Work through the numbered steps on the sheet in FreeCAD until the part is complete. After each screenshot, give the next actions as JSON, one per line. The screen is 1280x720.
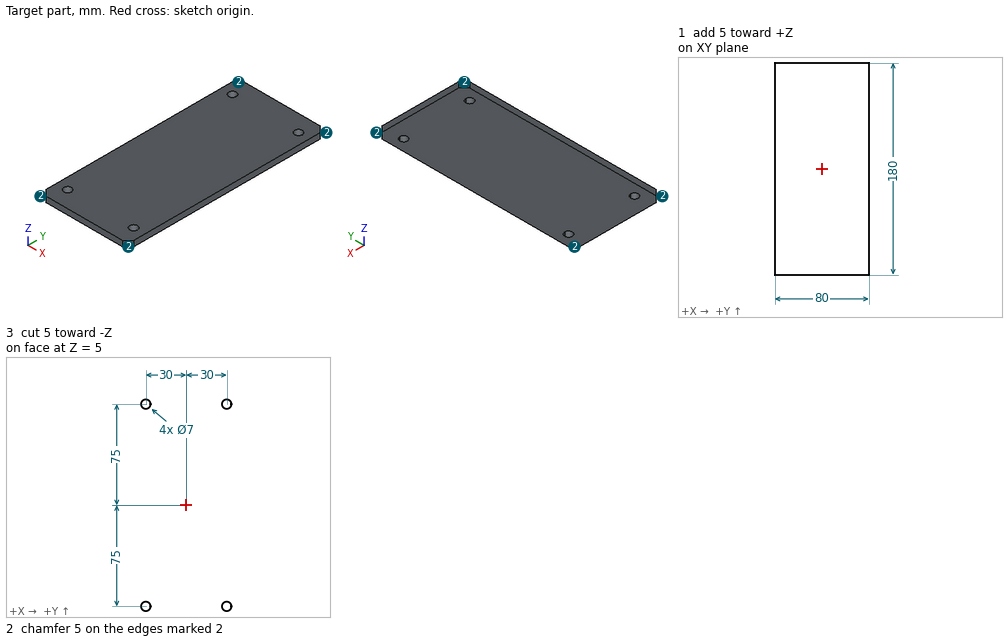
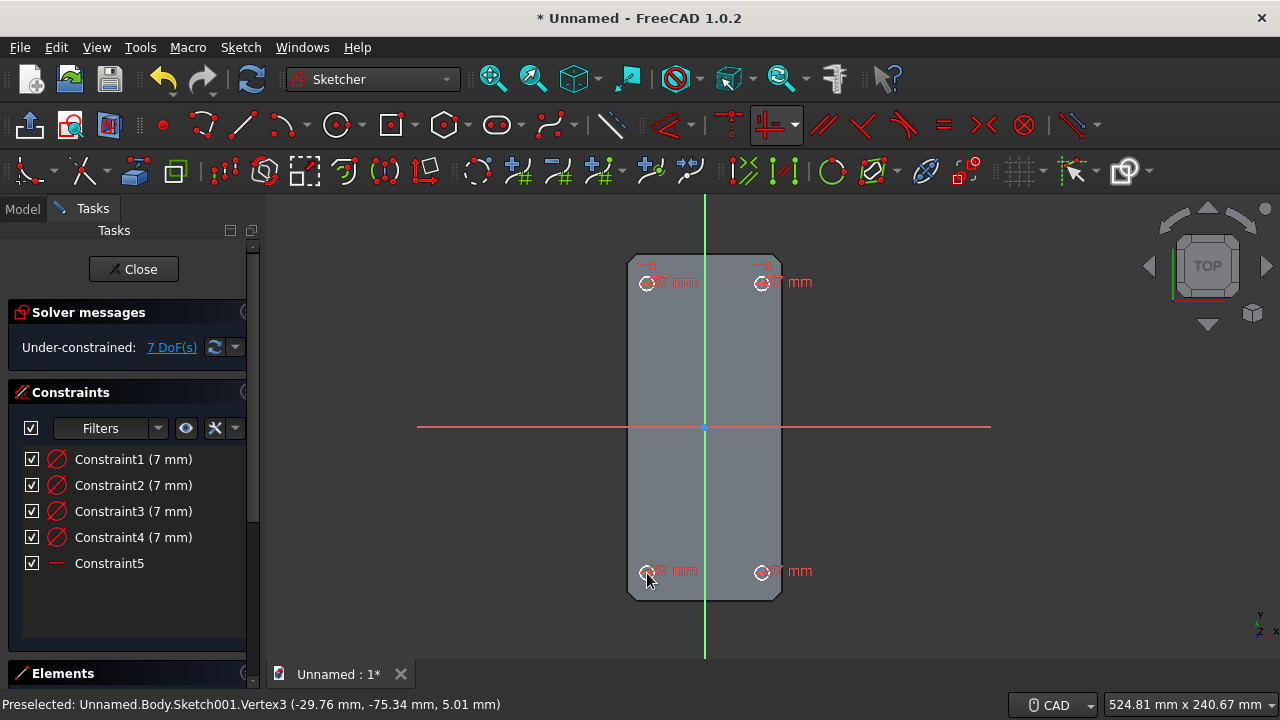
{"action": "left_click", "coordinate": [798, 126]}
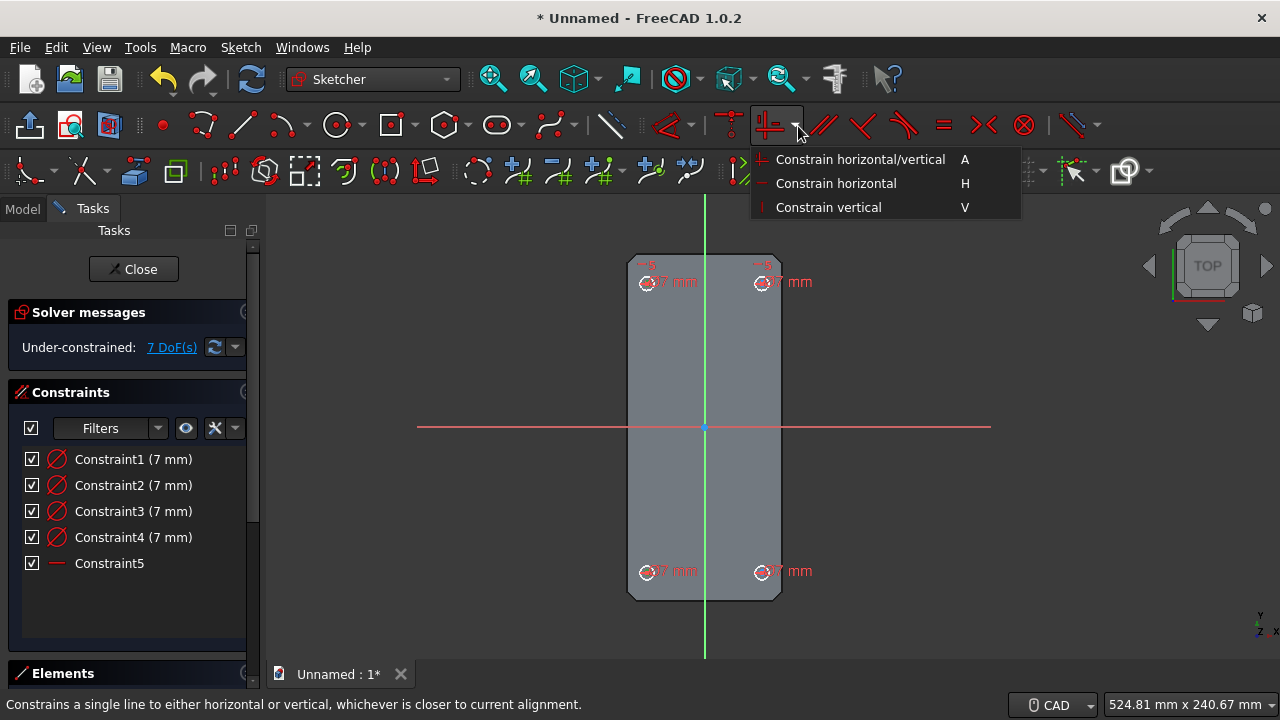
{"action": "left_click", "coordinate": [886, 207]}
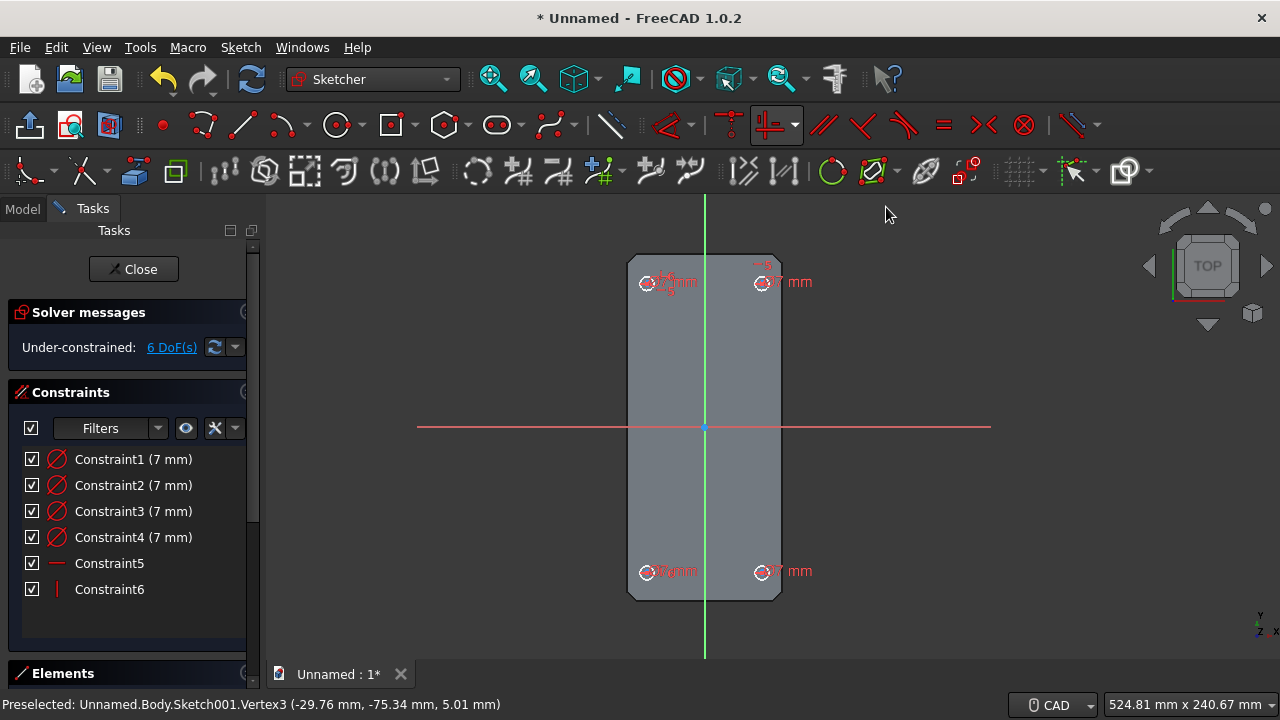
{"action": "left_click", "coordinate": [762, 284]}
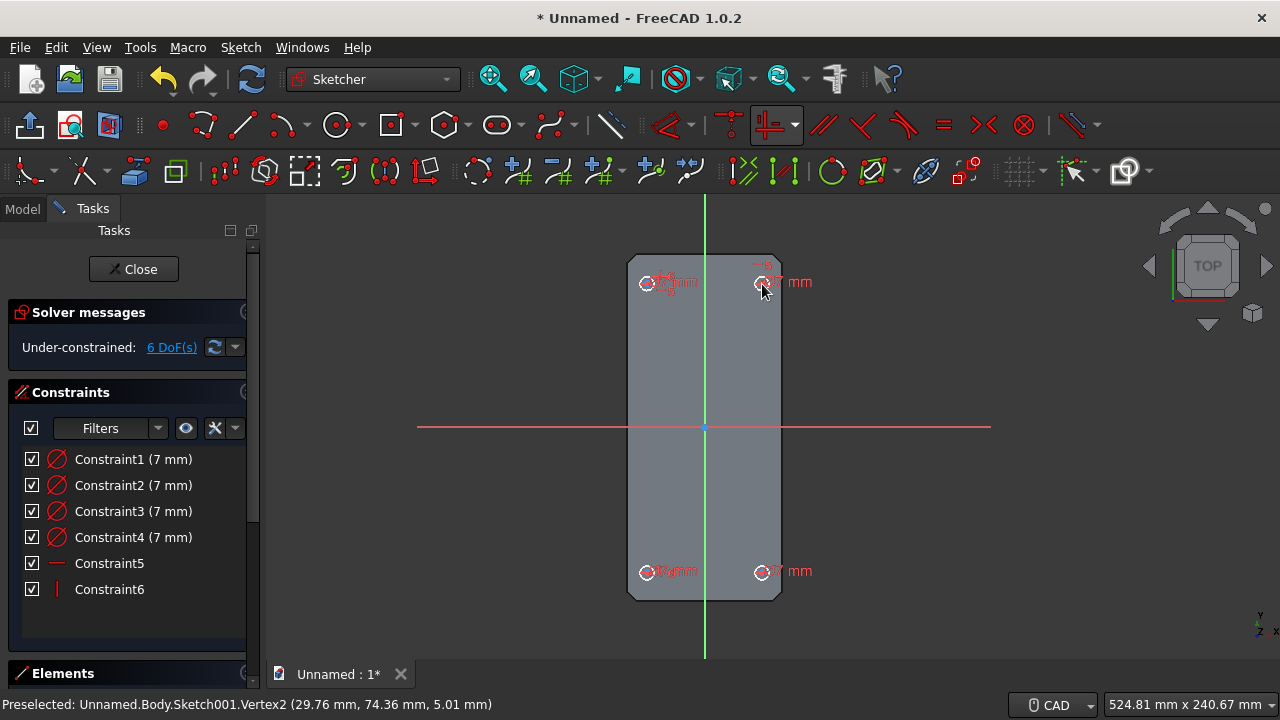
{"action": "left_click", "coordinate": [762, 573]}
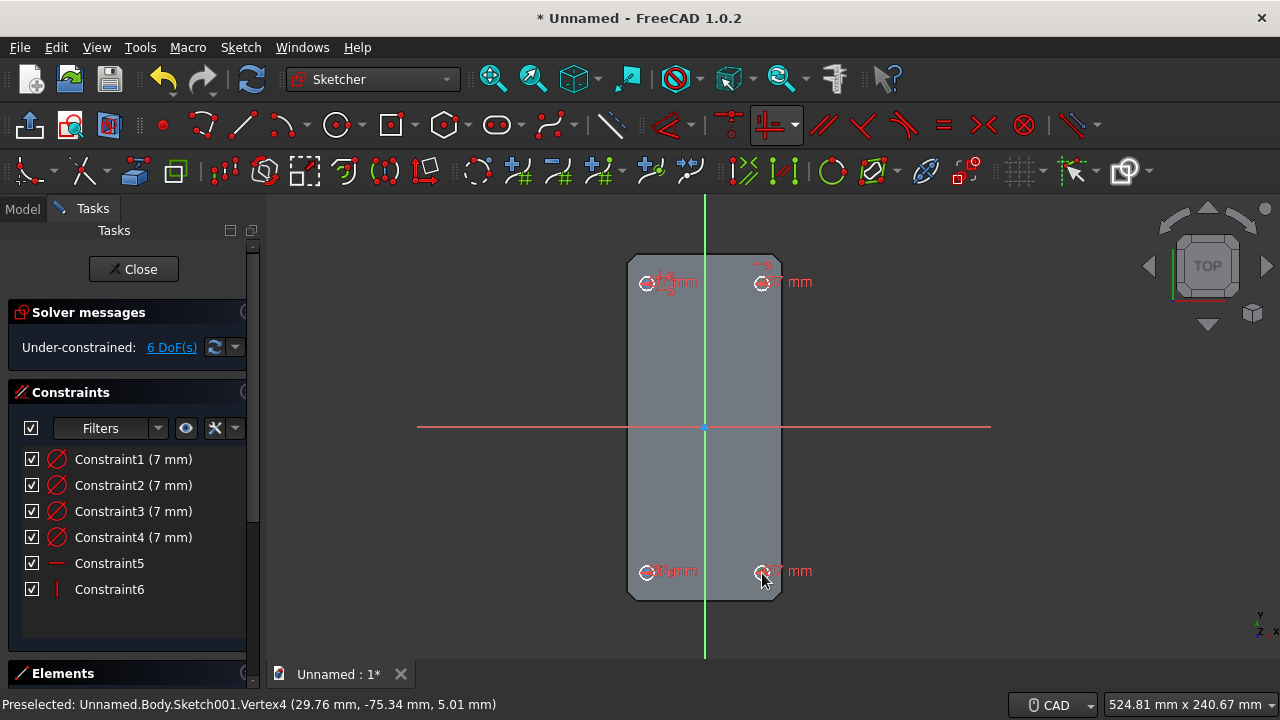
{"action": "left_click", "coordinate": [798, 126]}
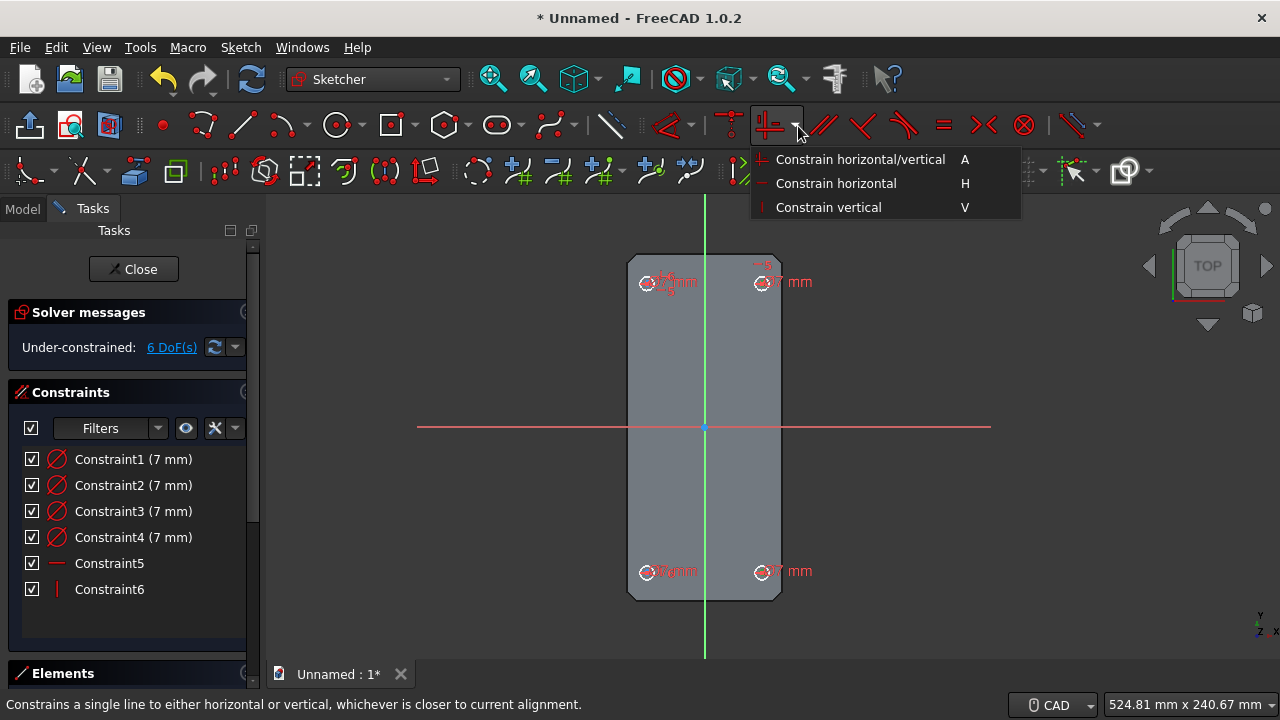
{"action": "left_click", "coordinate": [886, 207]}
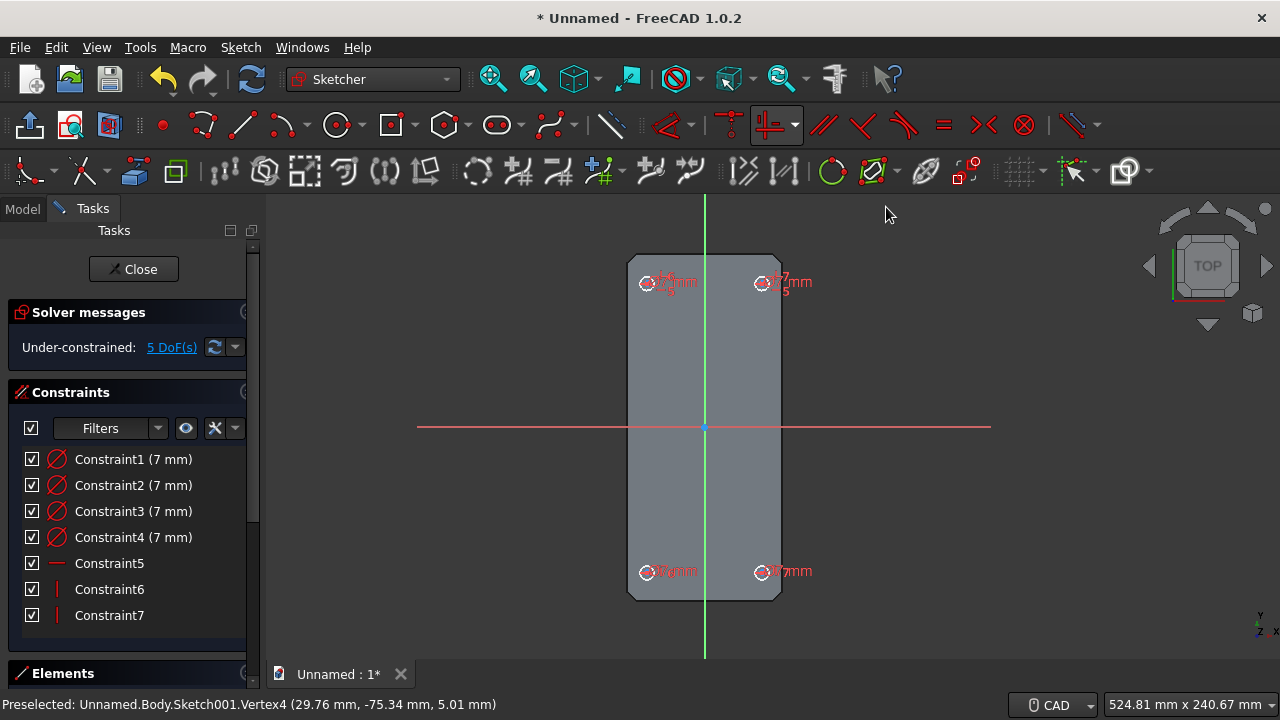
{"action": "left_click", "coordinate": [647, 573]}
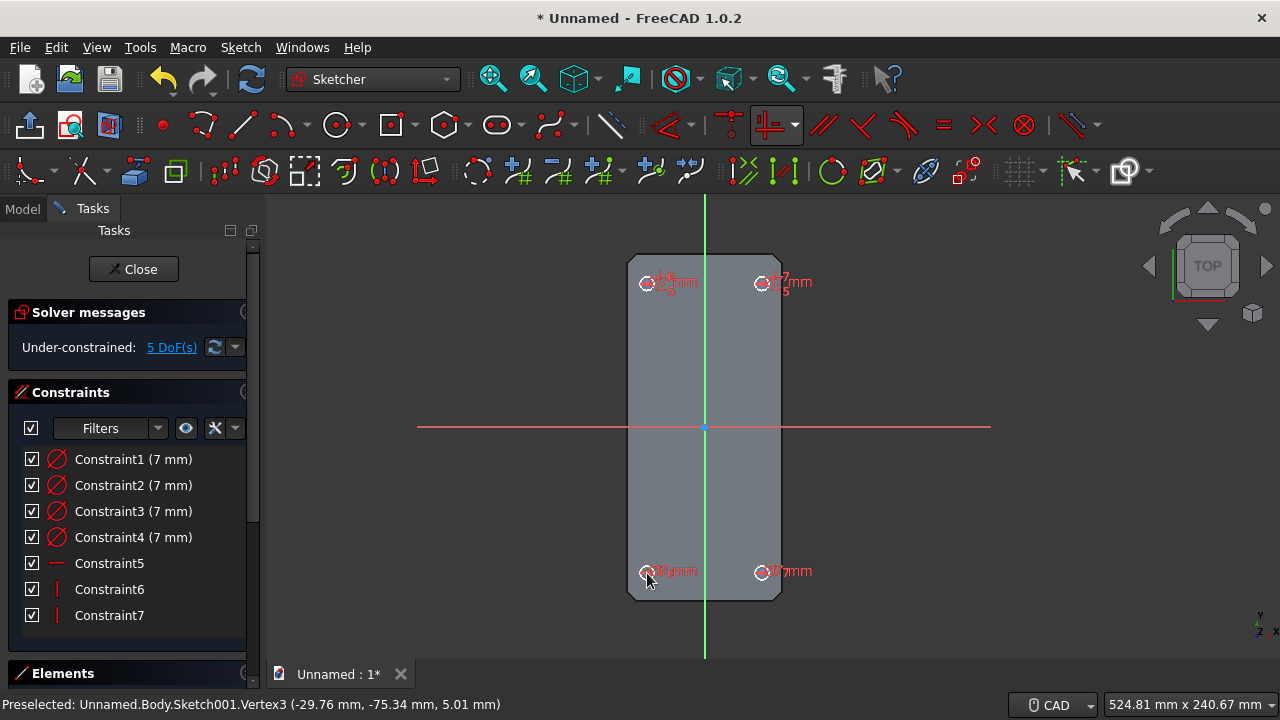
{"action": "left_click", "coordinate": [762, 573]}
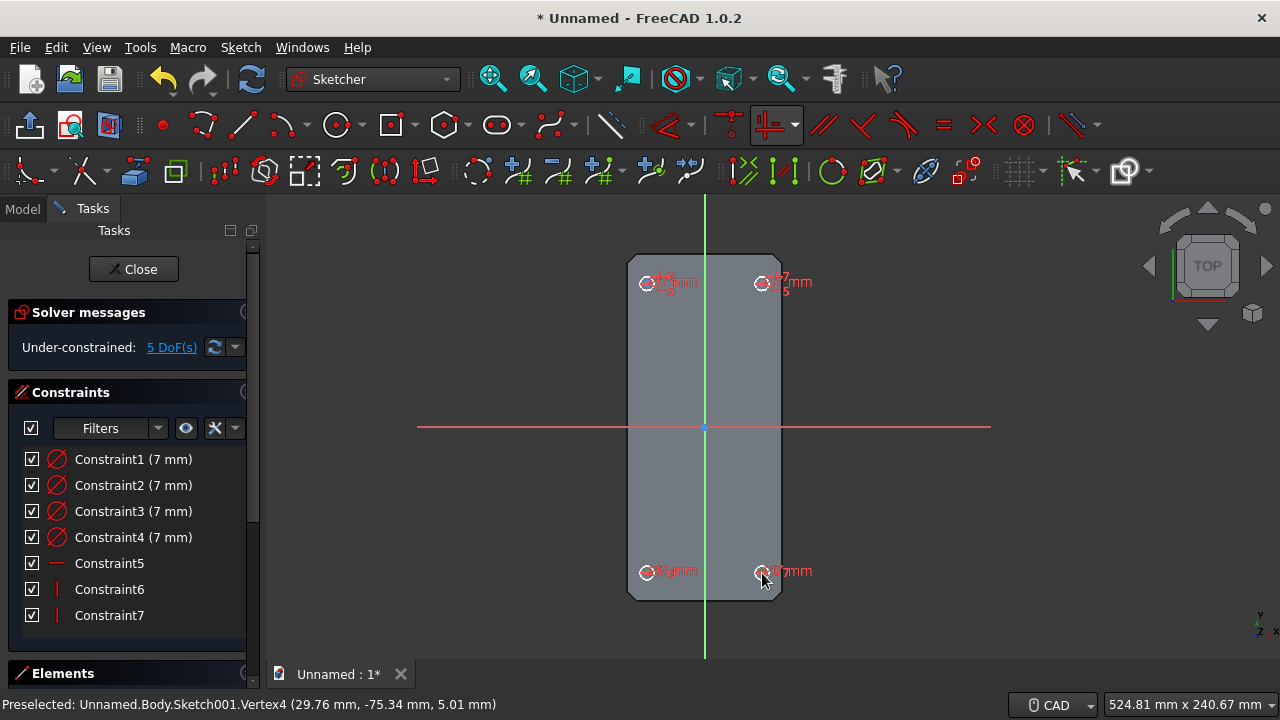
{"action": "key", "text": "h"}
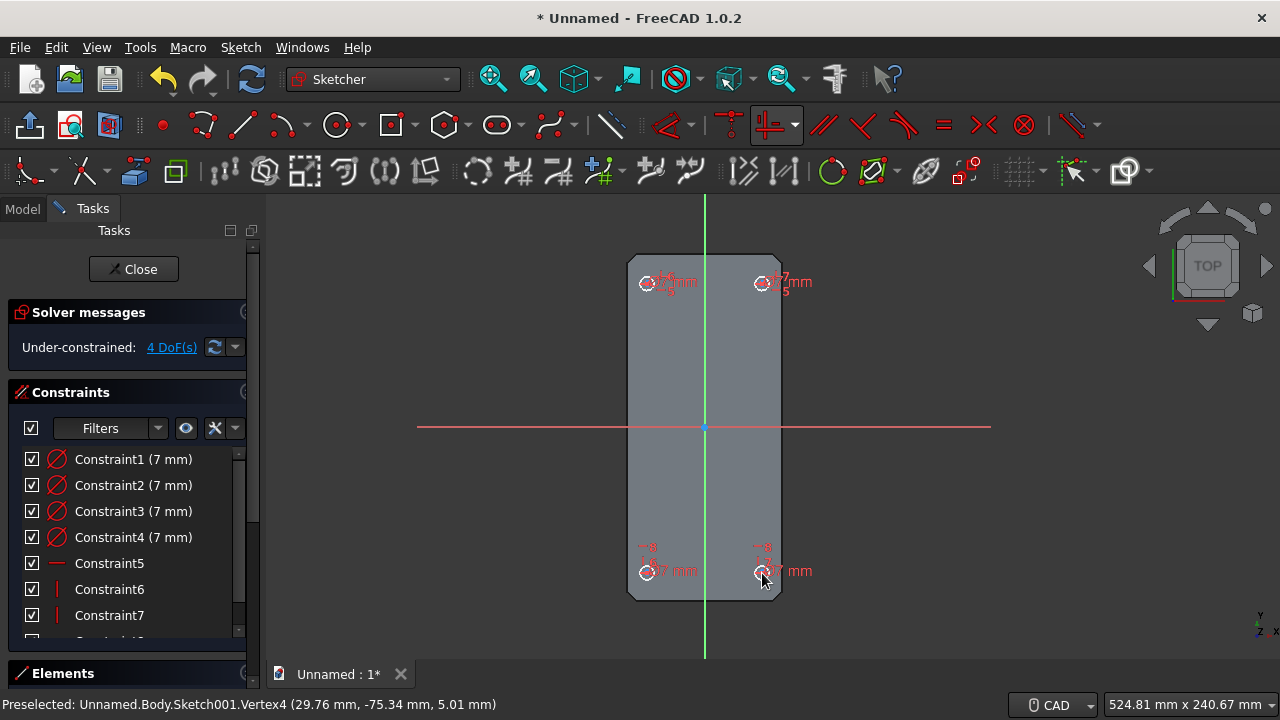
{"action": "left_click", "coordinate": [666, 126]}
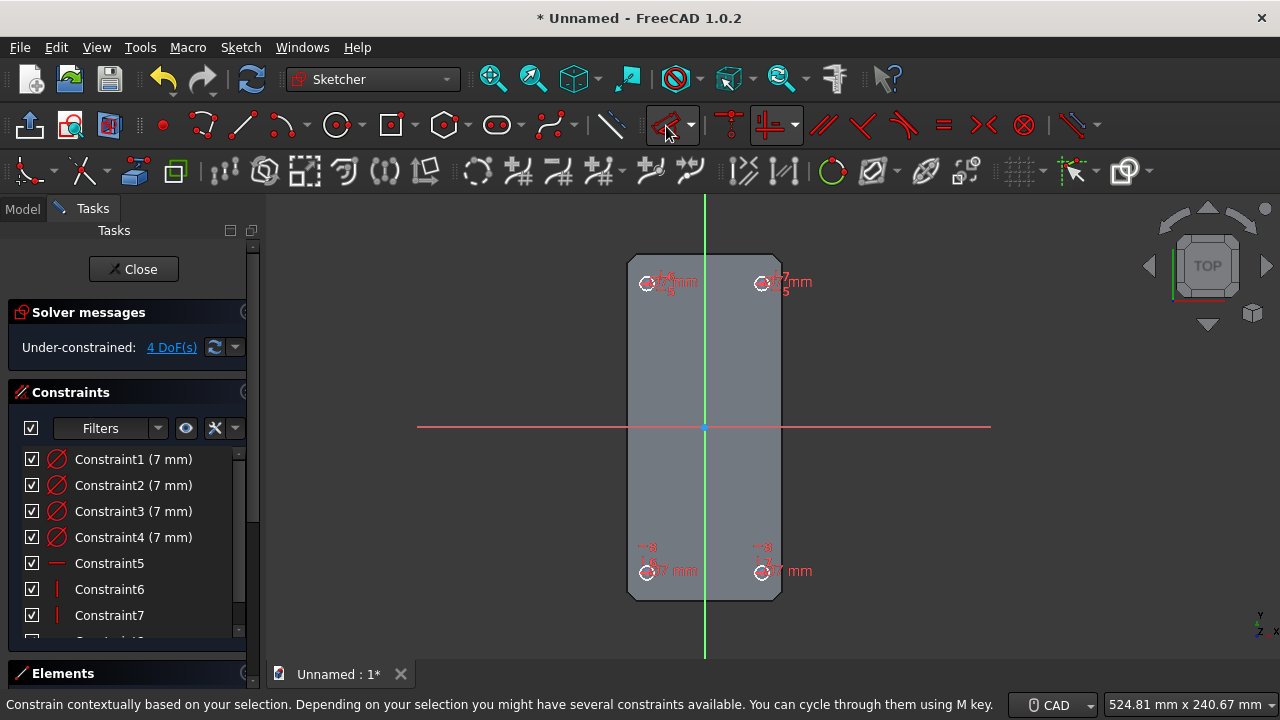
{"action": "left_click", "coordinate": [647, 284]}
{"action": "left_click", "coordinate": [676, 250]}